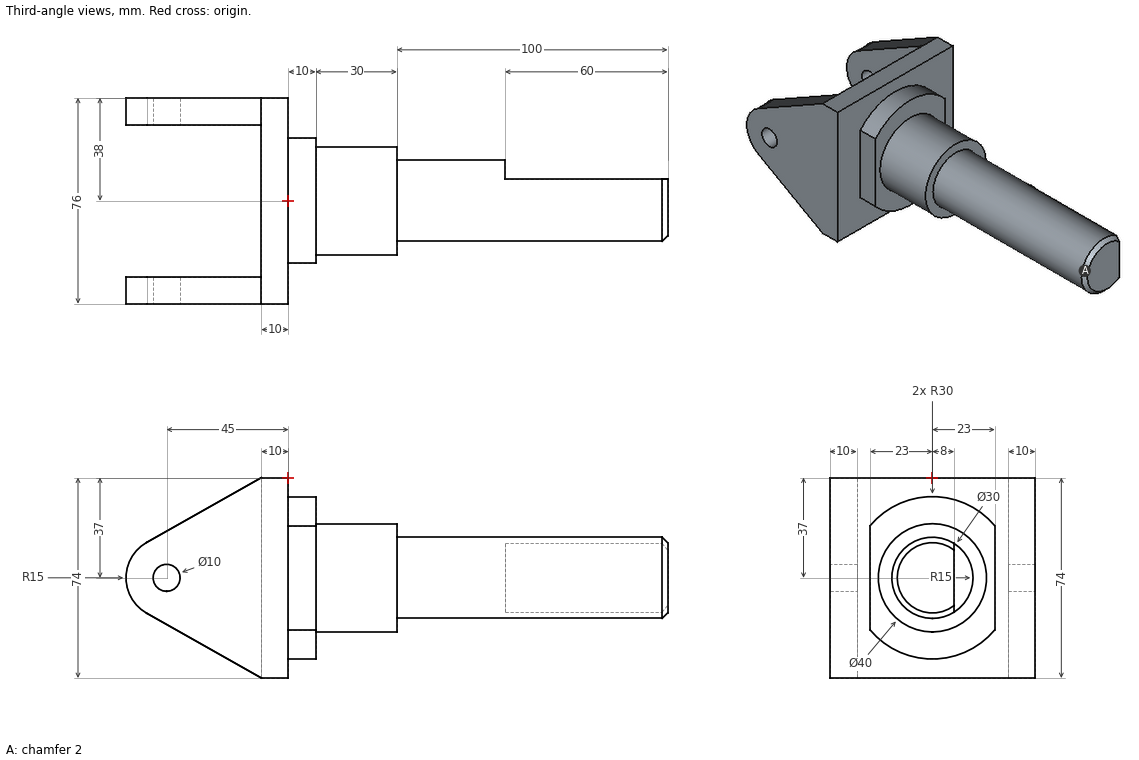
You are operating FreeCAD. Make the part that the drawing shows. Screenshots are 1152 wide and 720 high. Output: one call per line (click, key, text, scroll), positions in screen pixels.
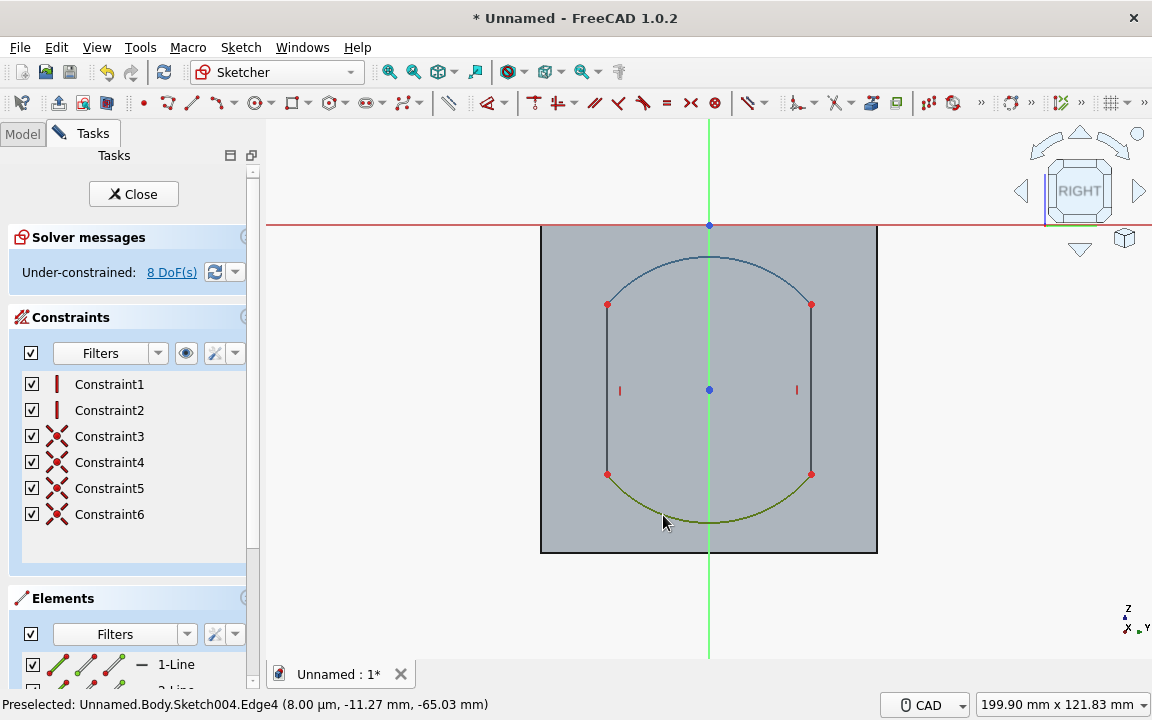
key(c)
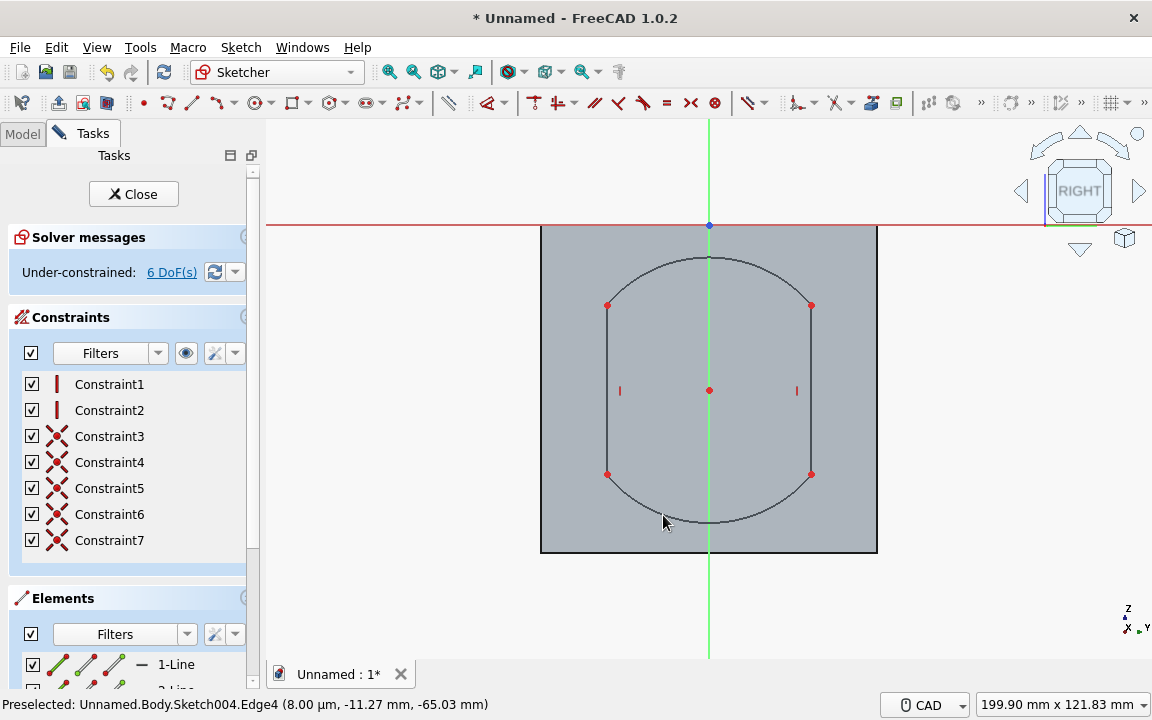
click(755, 265)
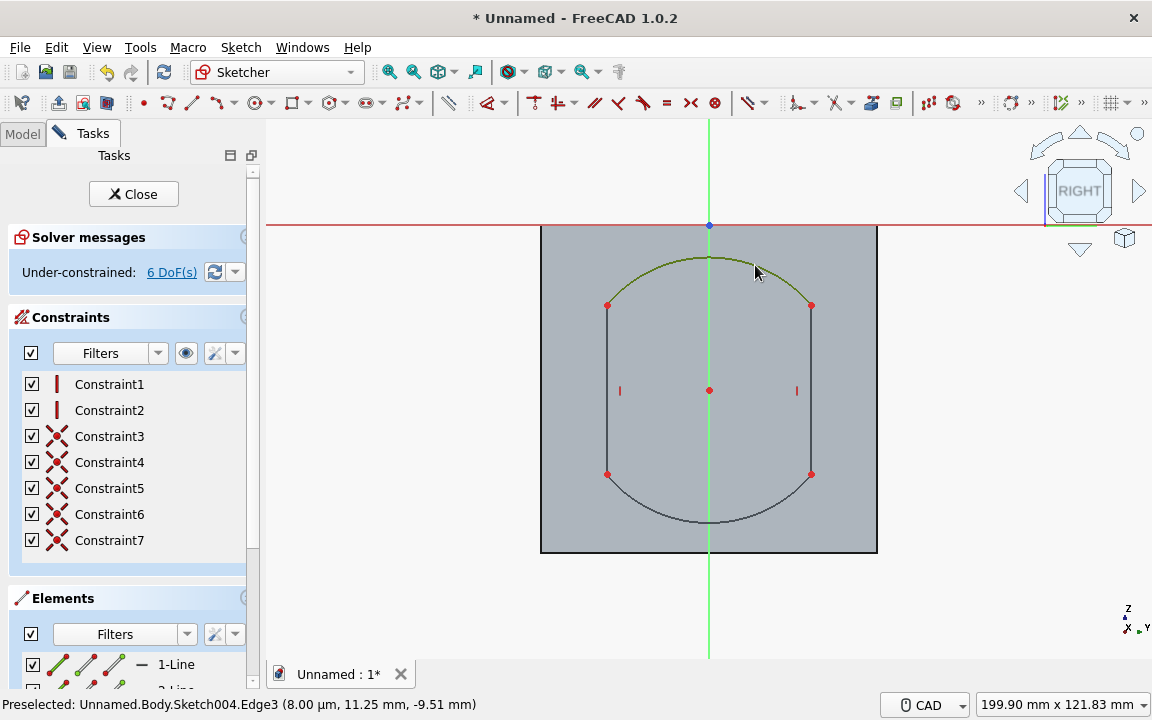
click(663, 515)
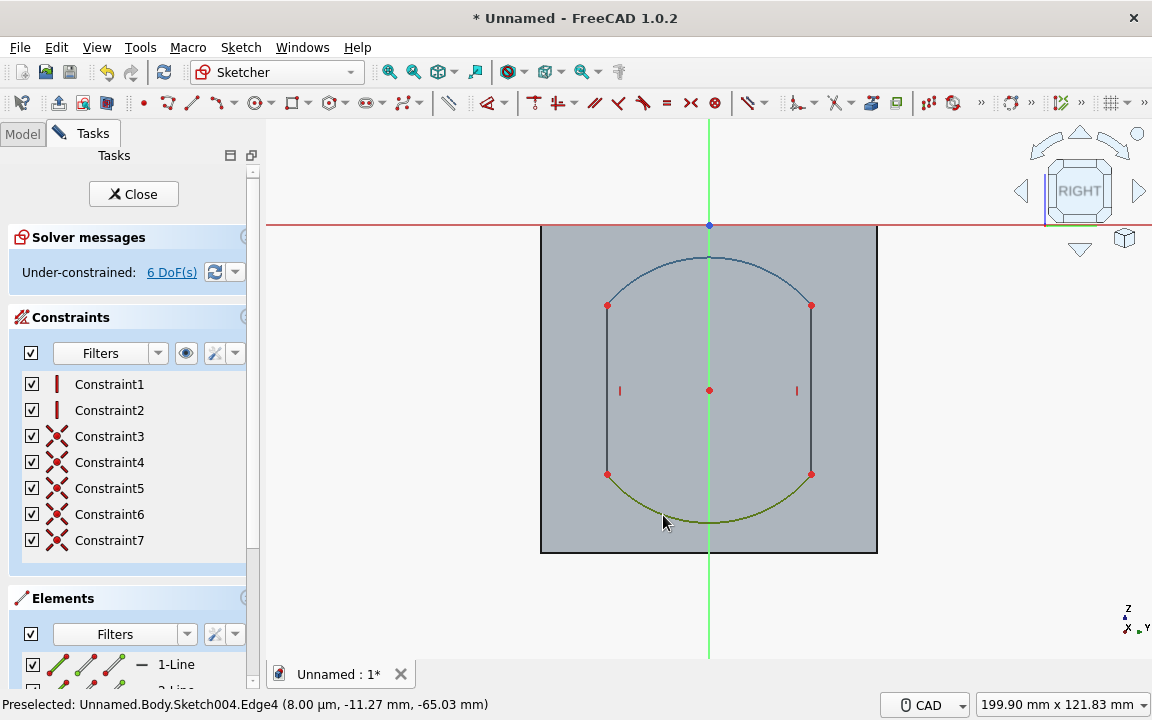
click(668, 104)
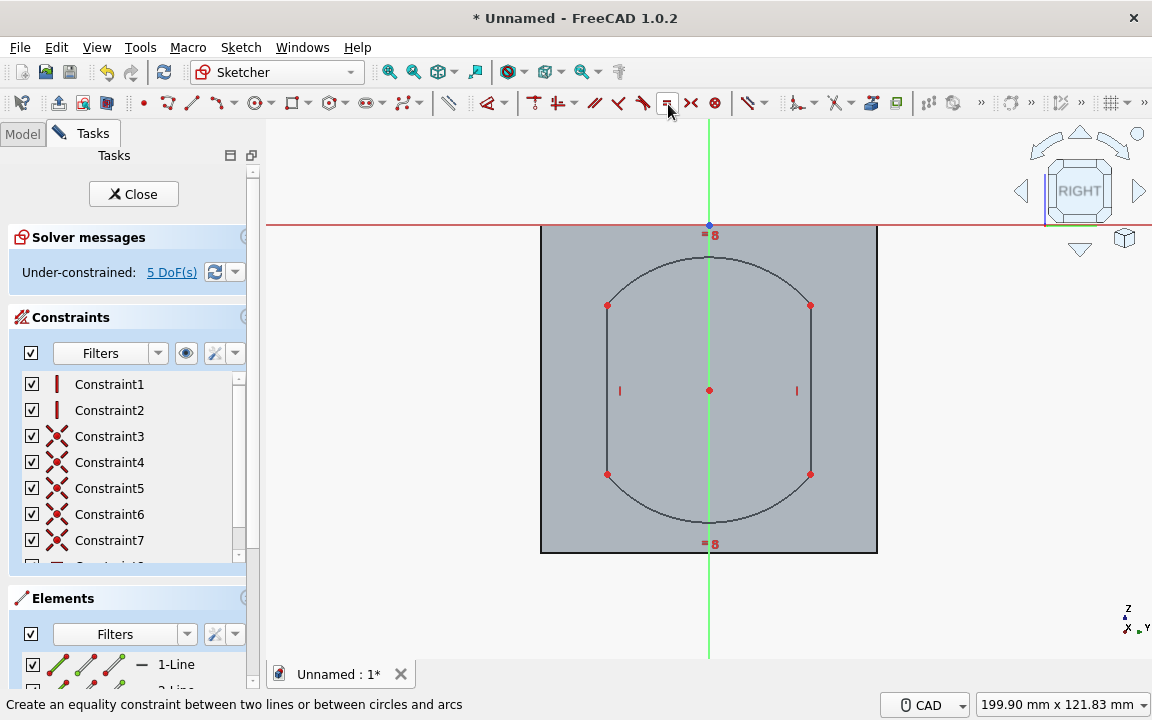
click(709, 390)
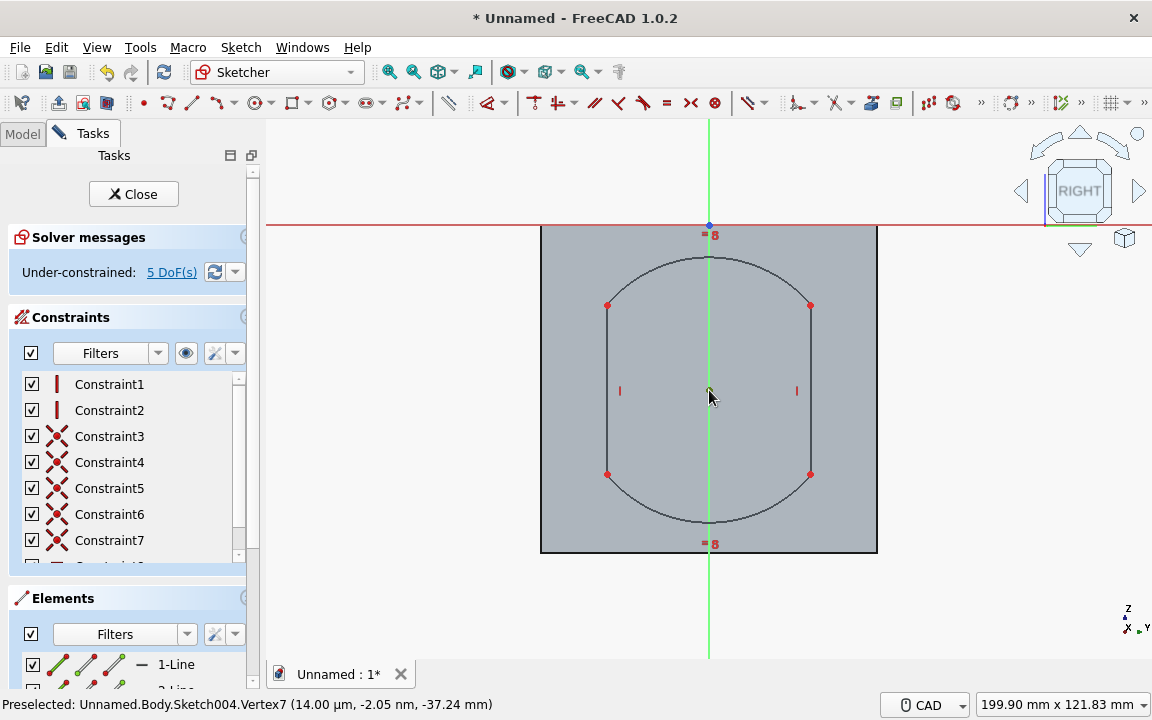
click(709, 596)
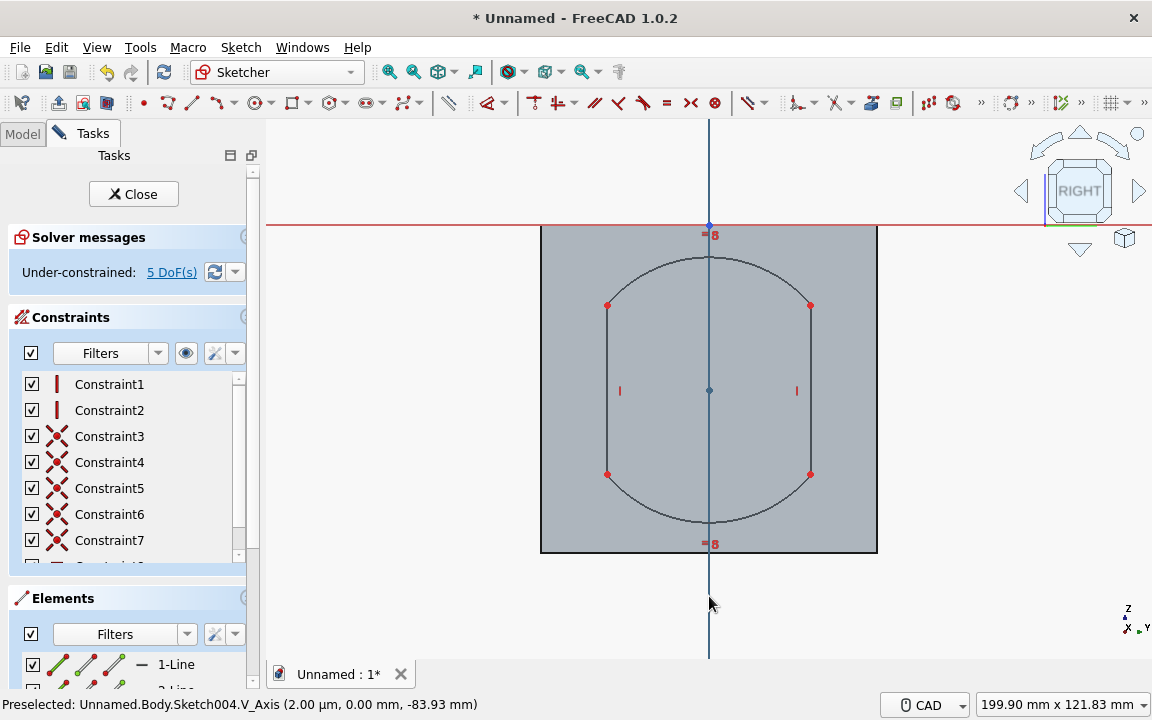
key(c)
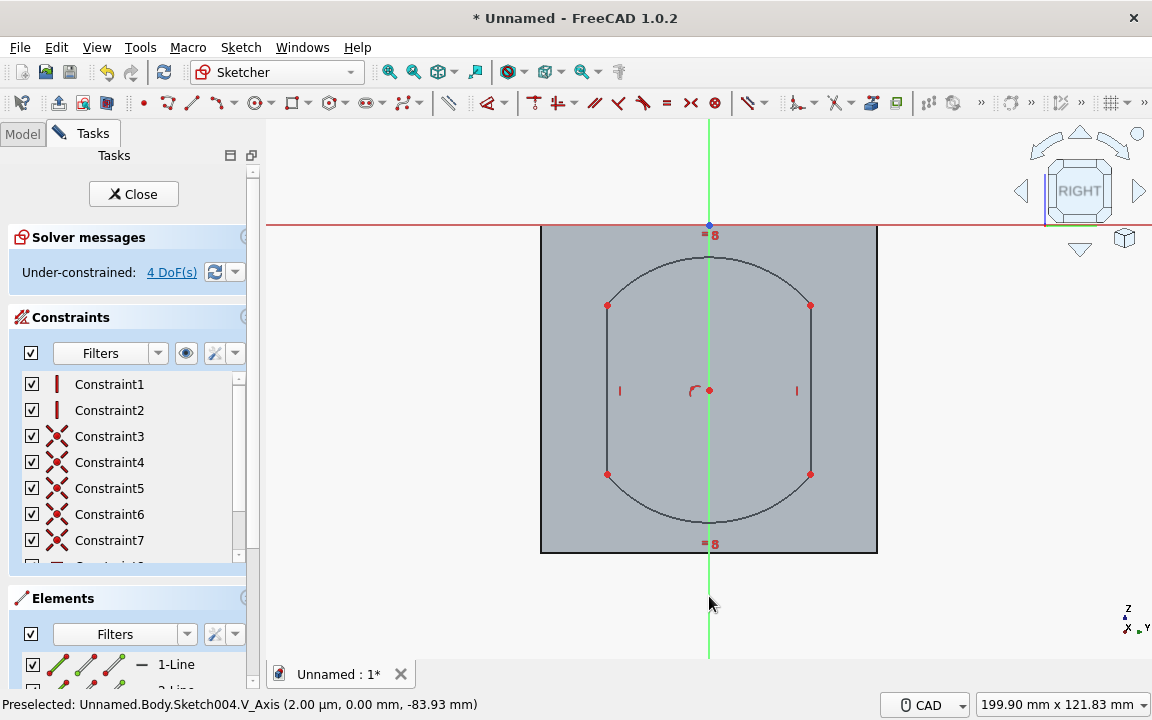
click(488, 104)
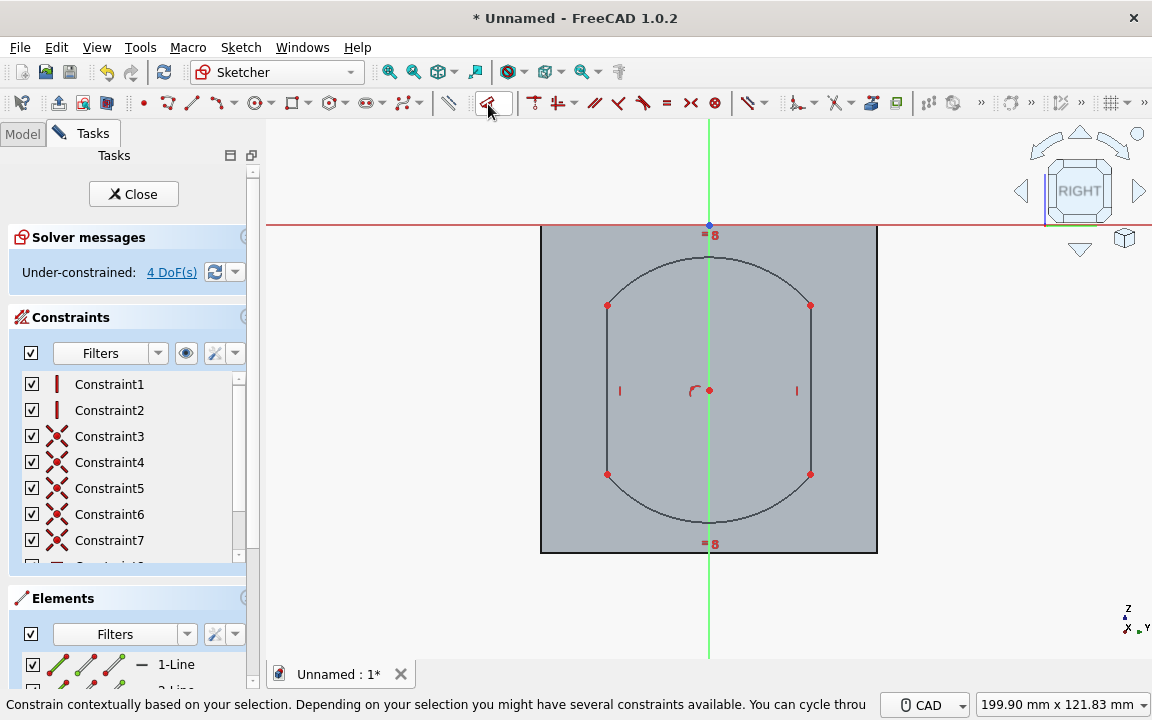
click(755, 265)
click(833, 281)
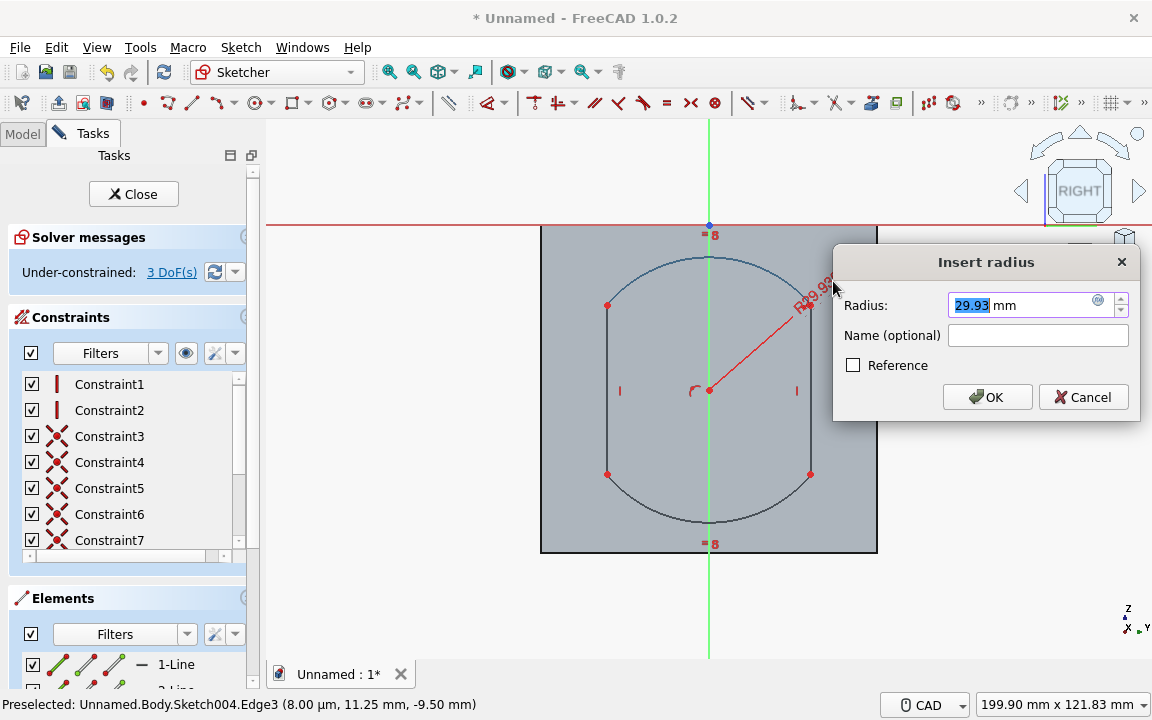
text(30)
key(Return)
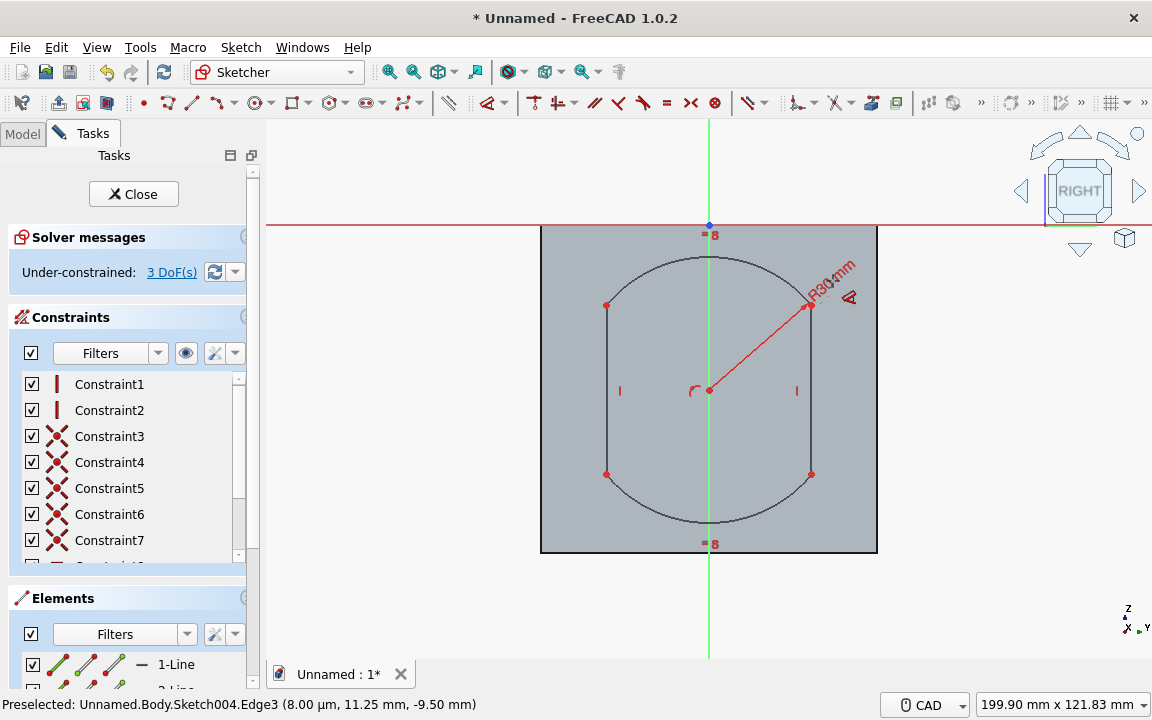
click(811, 475)
click(760, 191)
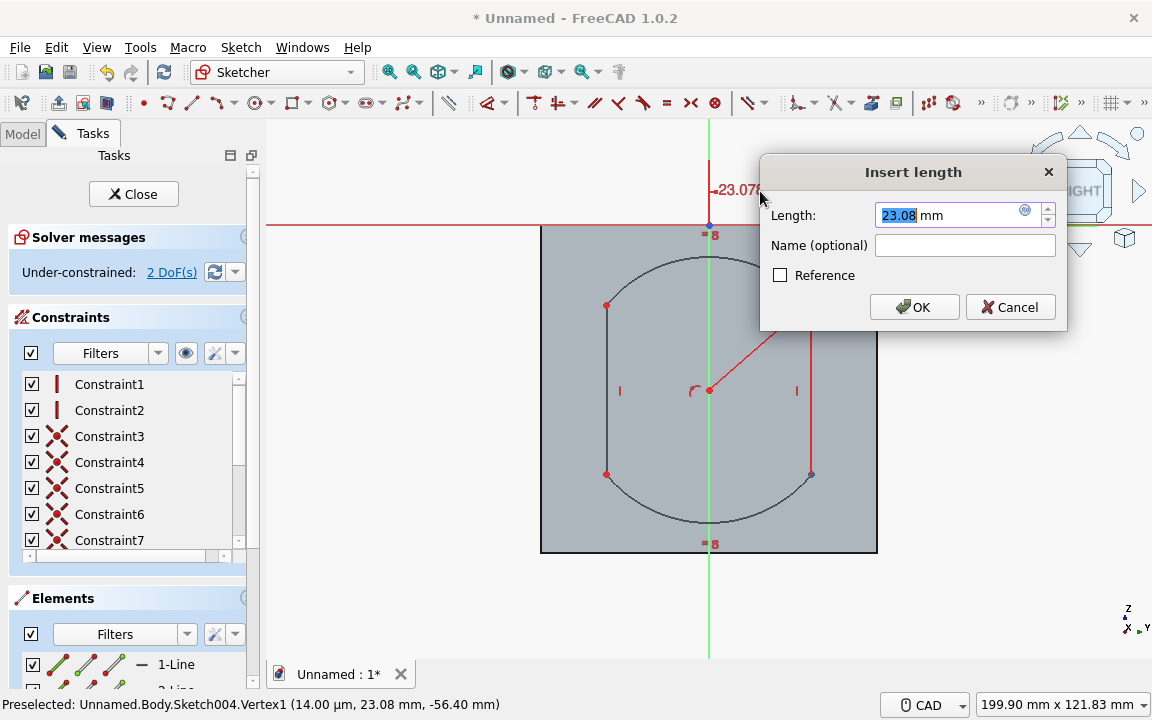
text(23)
key(Return)